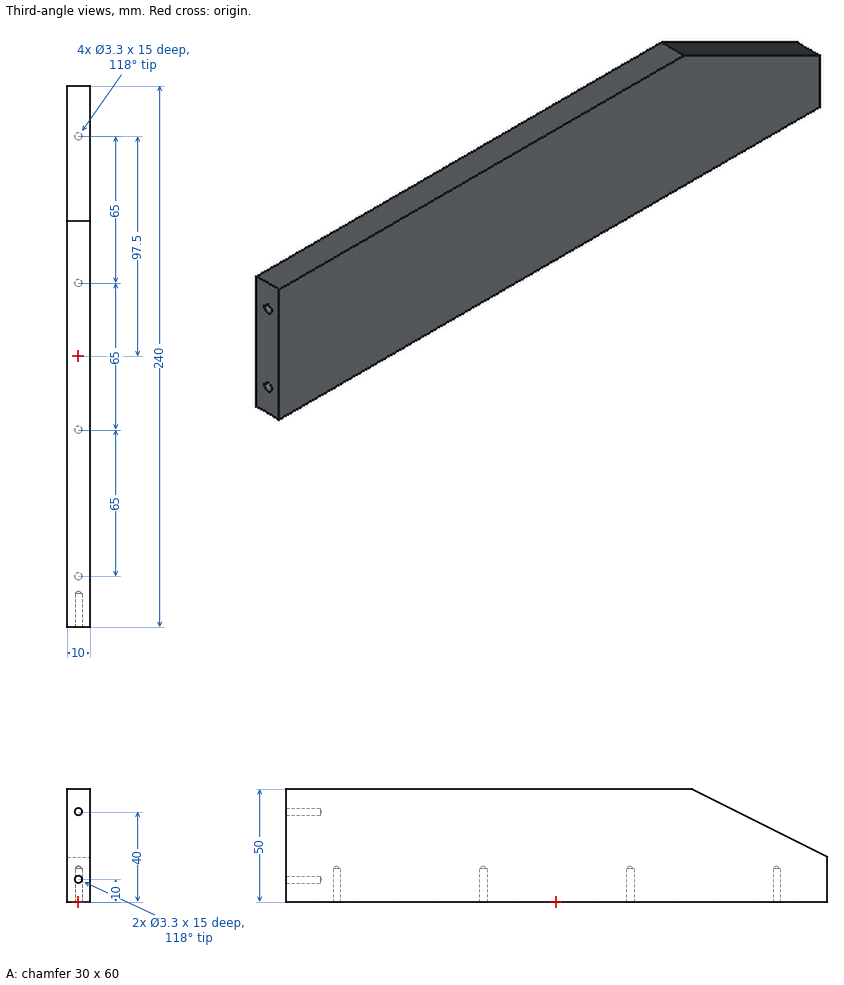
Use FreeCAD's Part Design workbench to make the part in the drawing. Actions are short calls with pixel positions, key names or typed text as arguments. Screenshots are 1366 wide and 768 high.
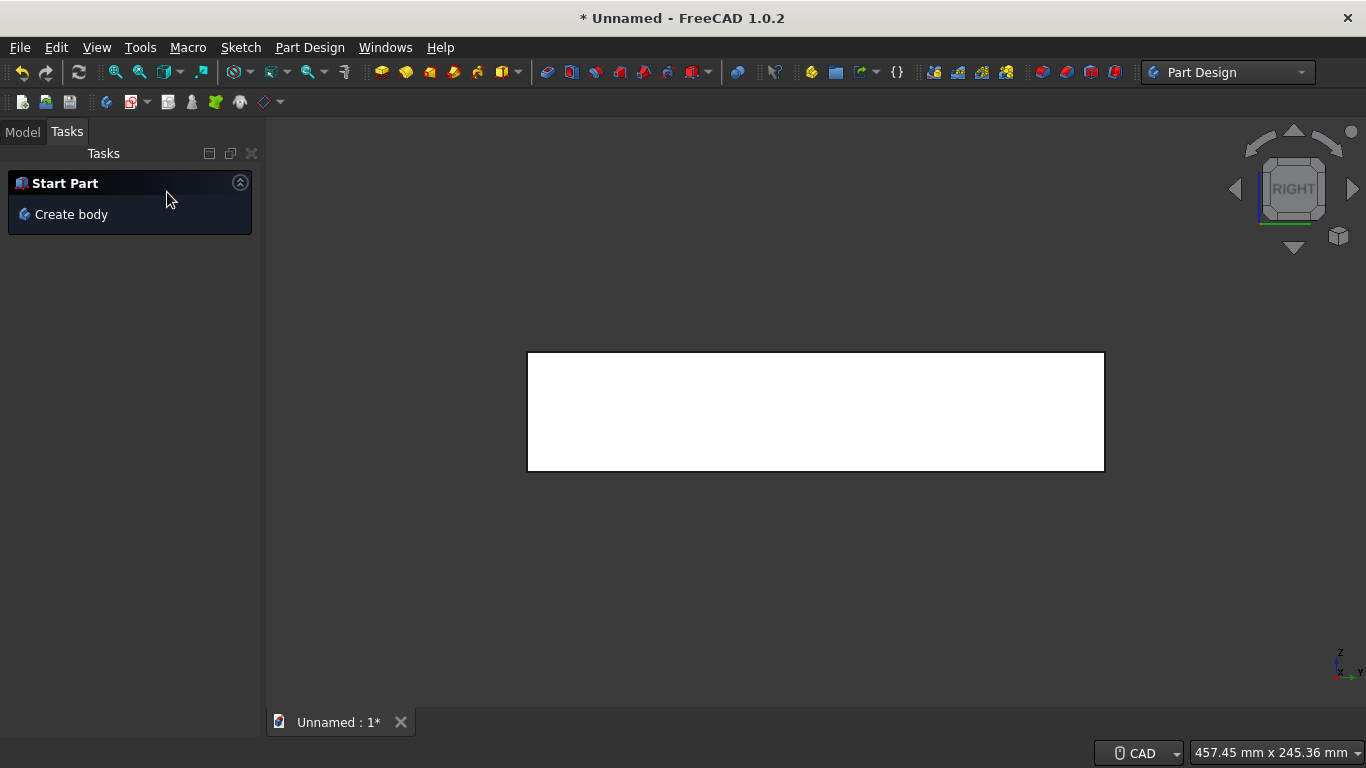
key(5)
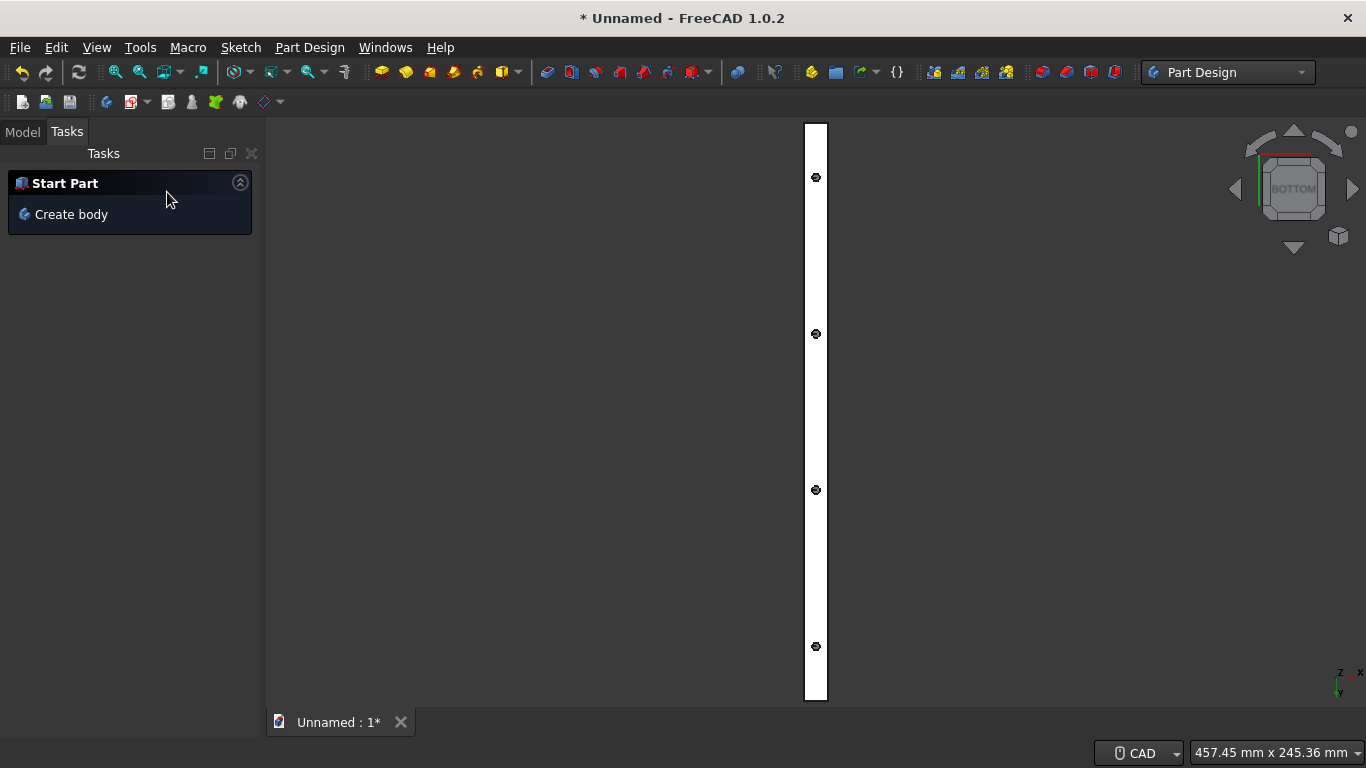
key(4)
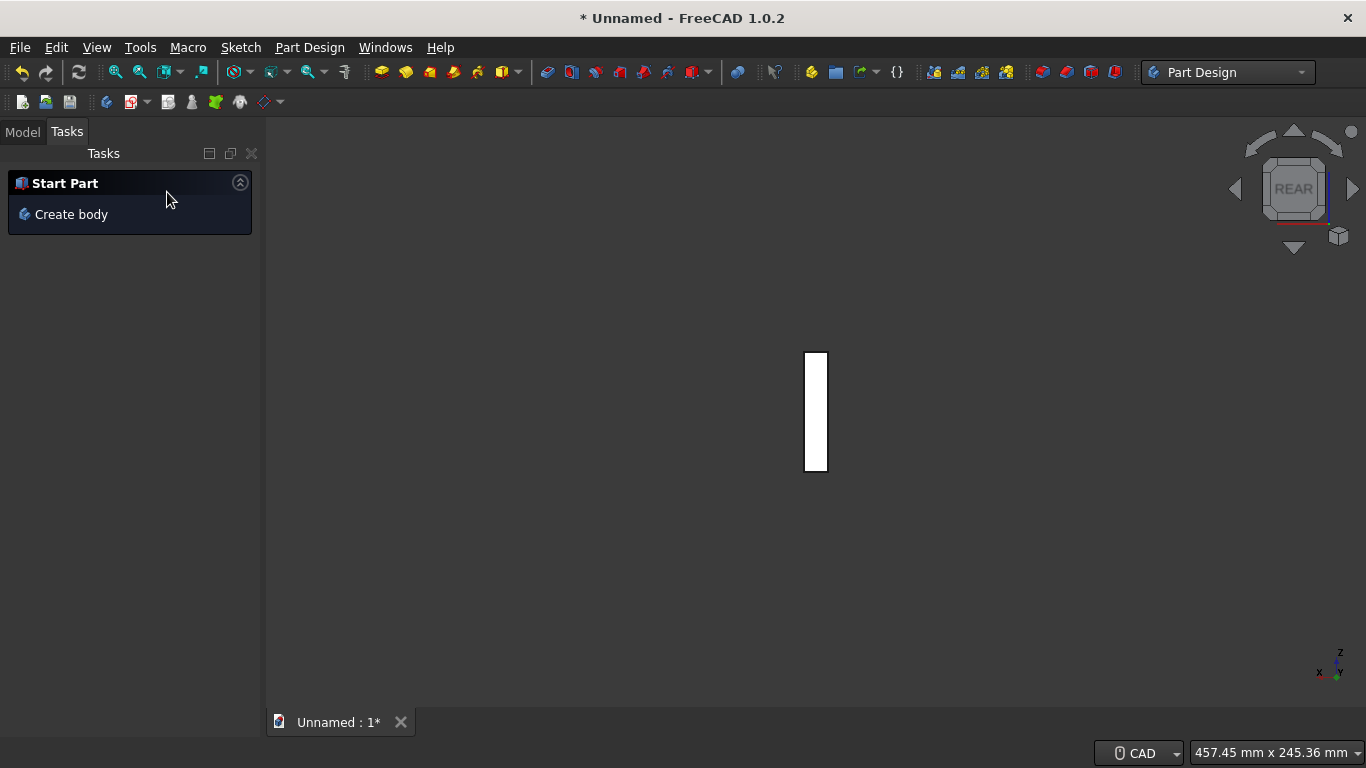
click(116, 72)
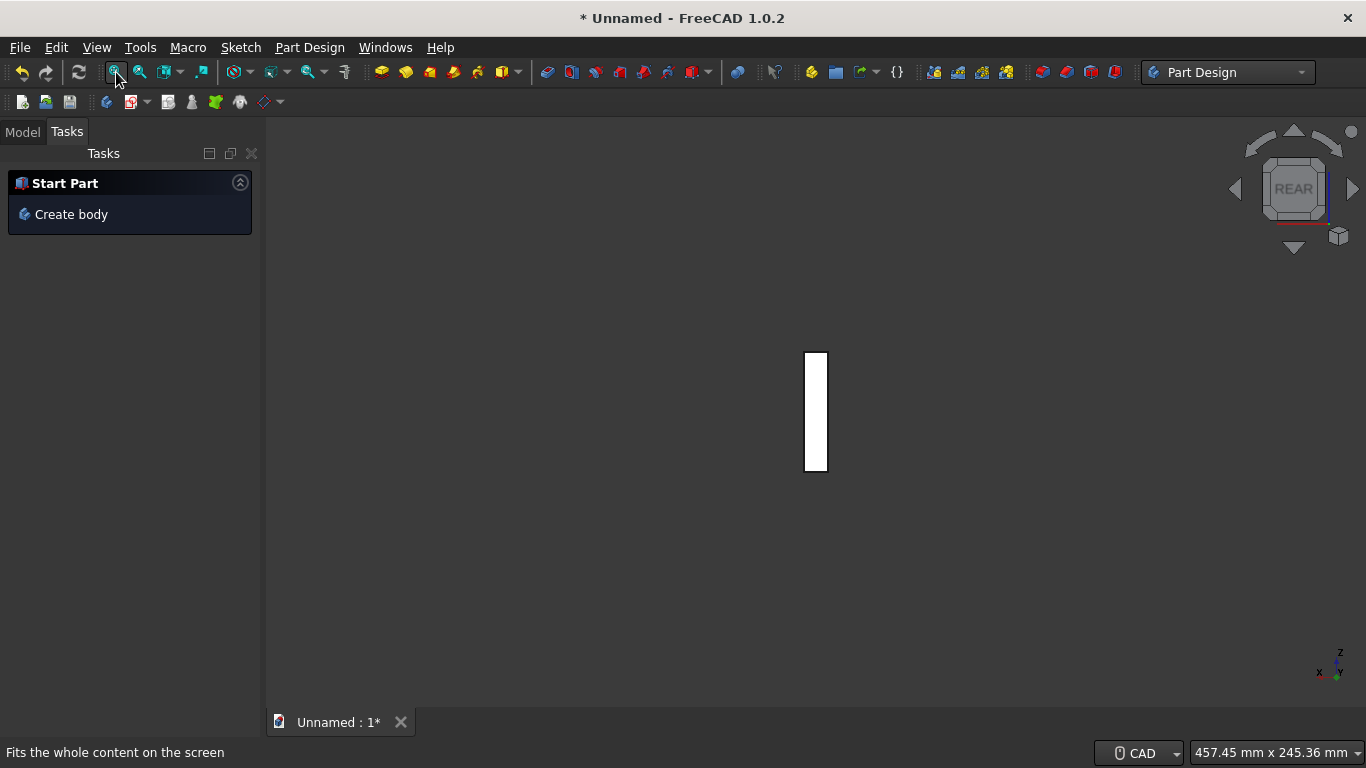
click(816, 351)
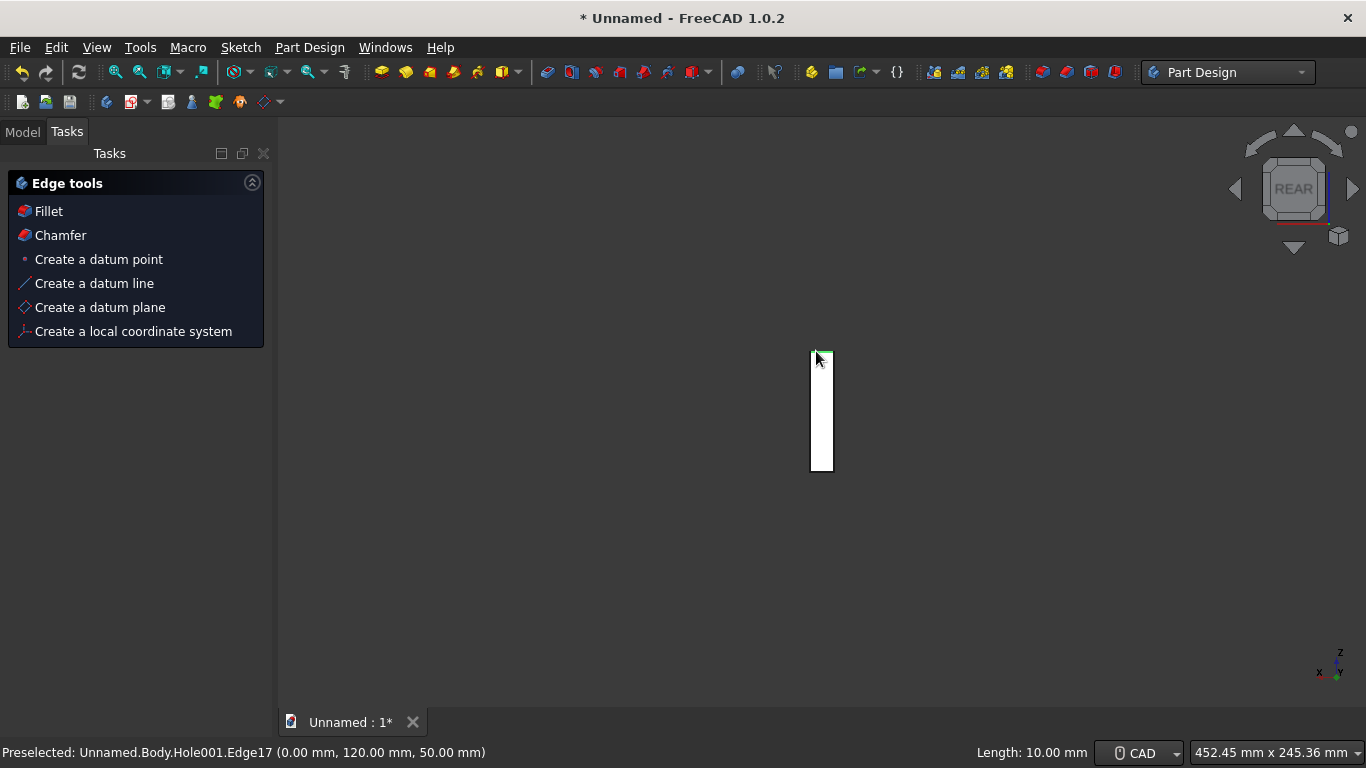
click(1068, 72)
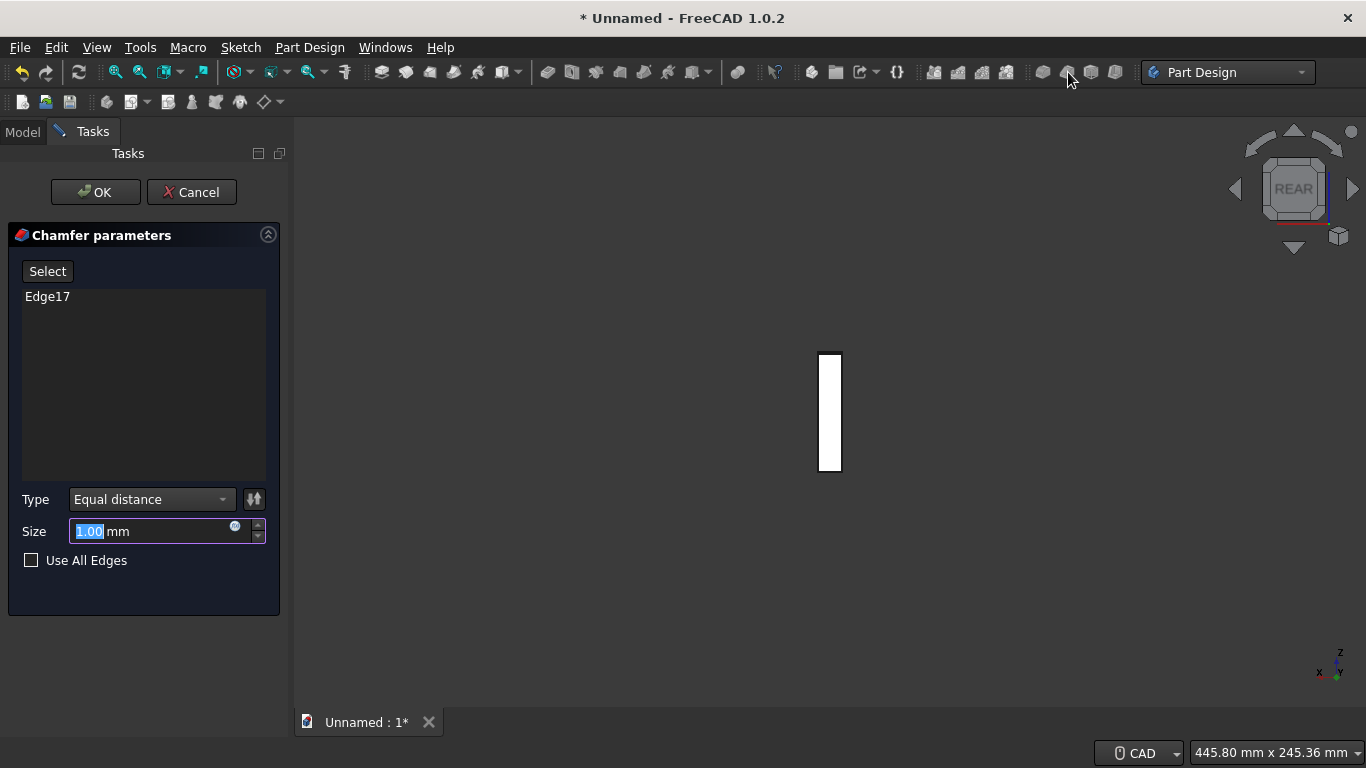
text(30)
key(Tab)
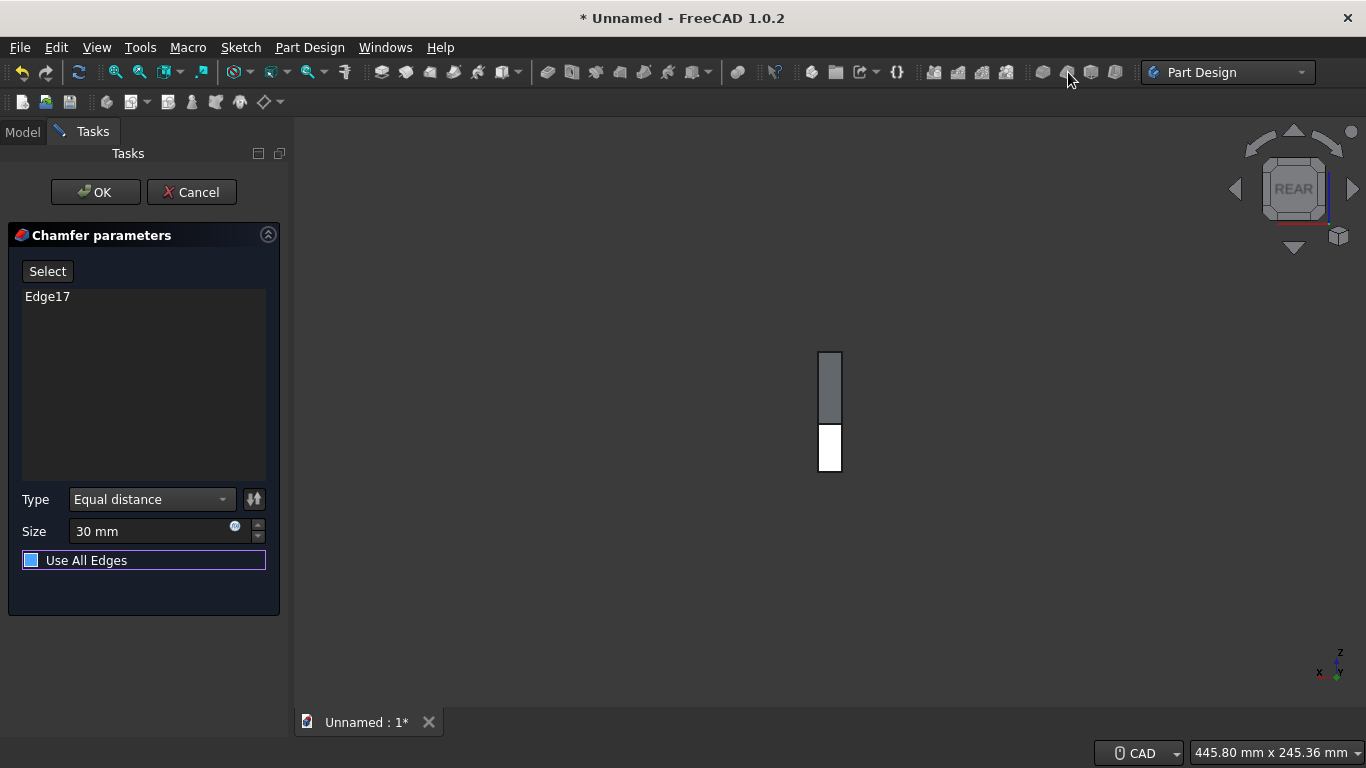
click(153, 500)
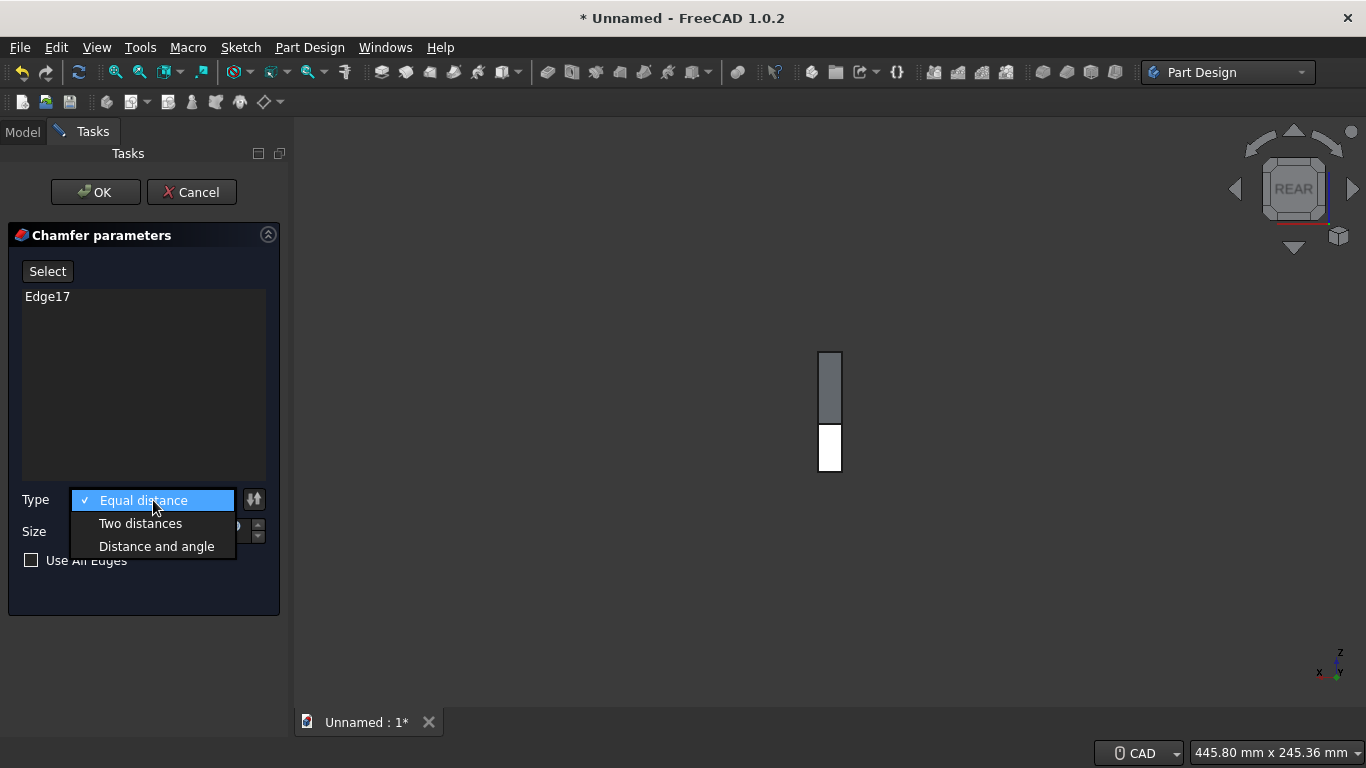
click(152, 524)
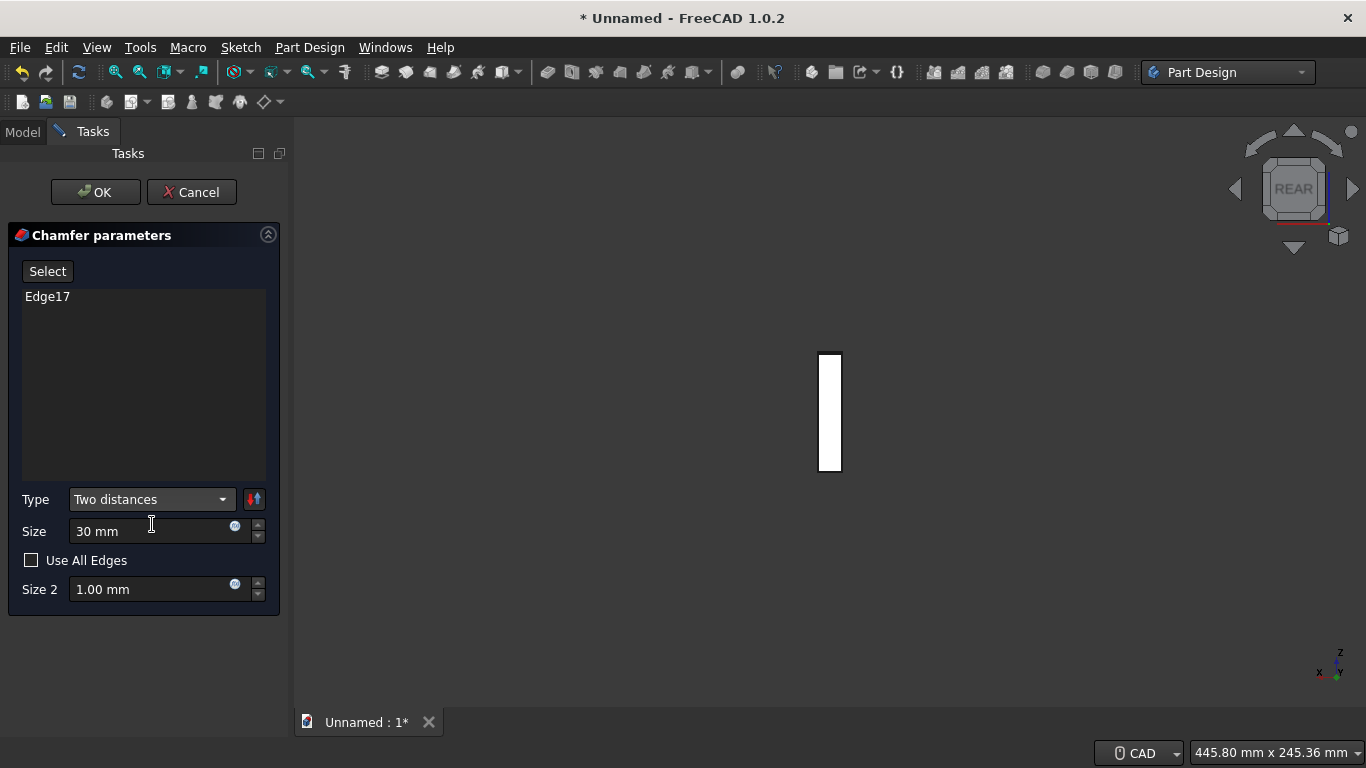
triple_click(160, 589)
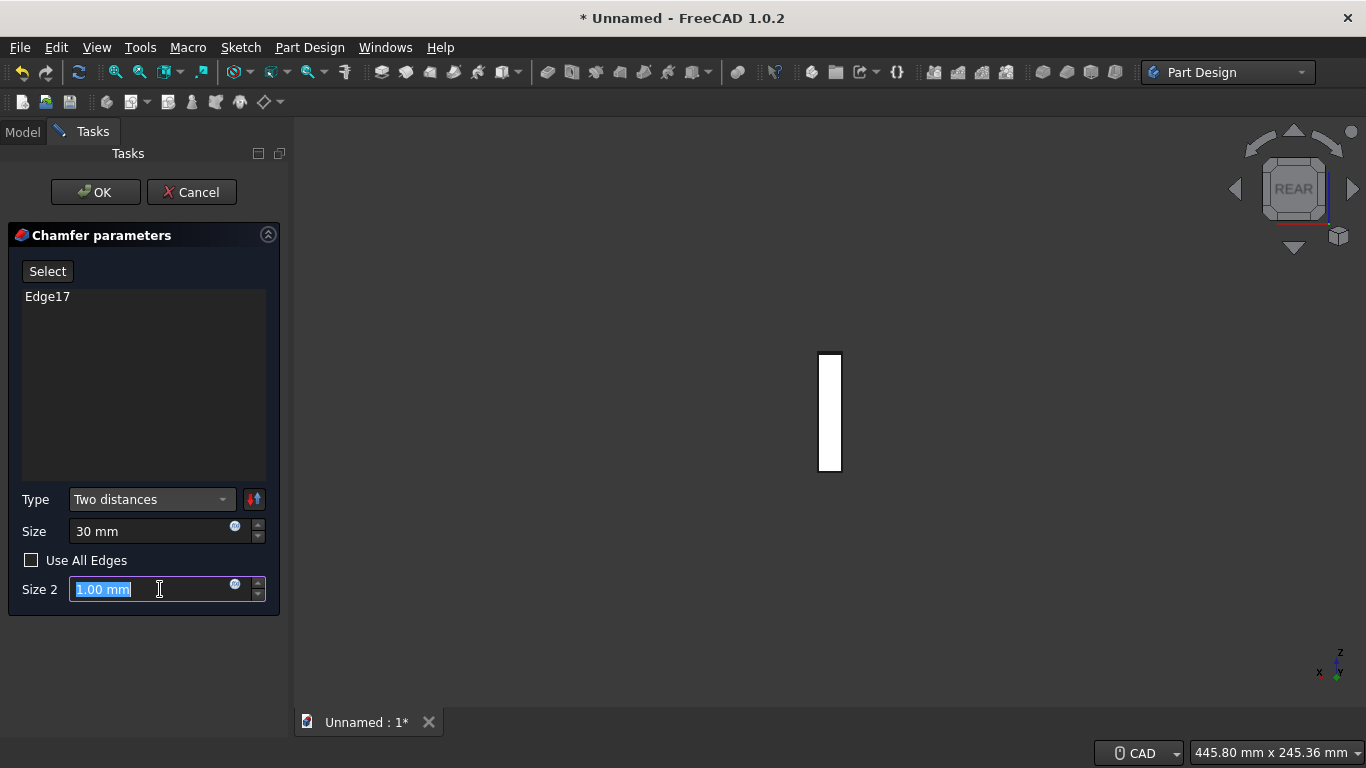
text(60)
key(Tab)